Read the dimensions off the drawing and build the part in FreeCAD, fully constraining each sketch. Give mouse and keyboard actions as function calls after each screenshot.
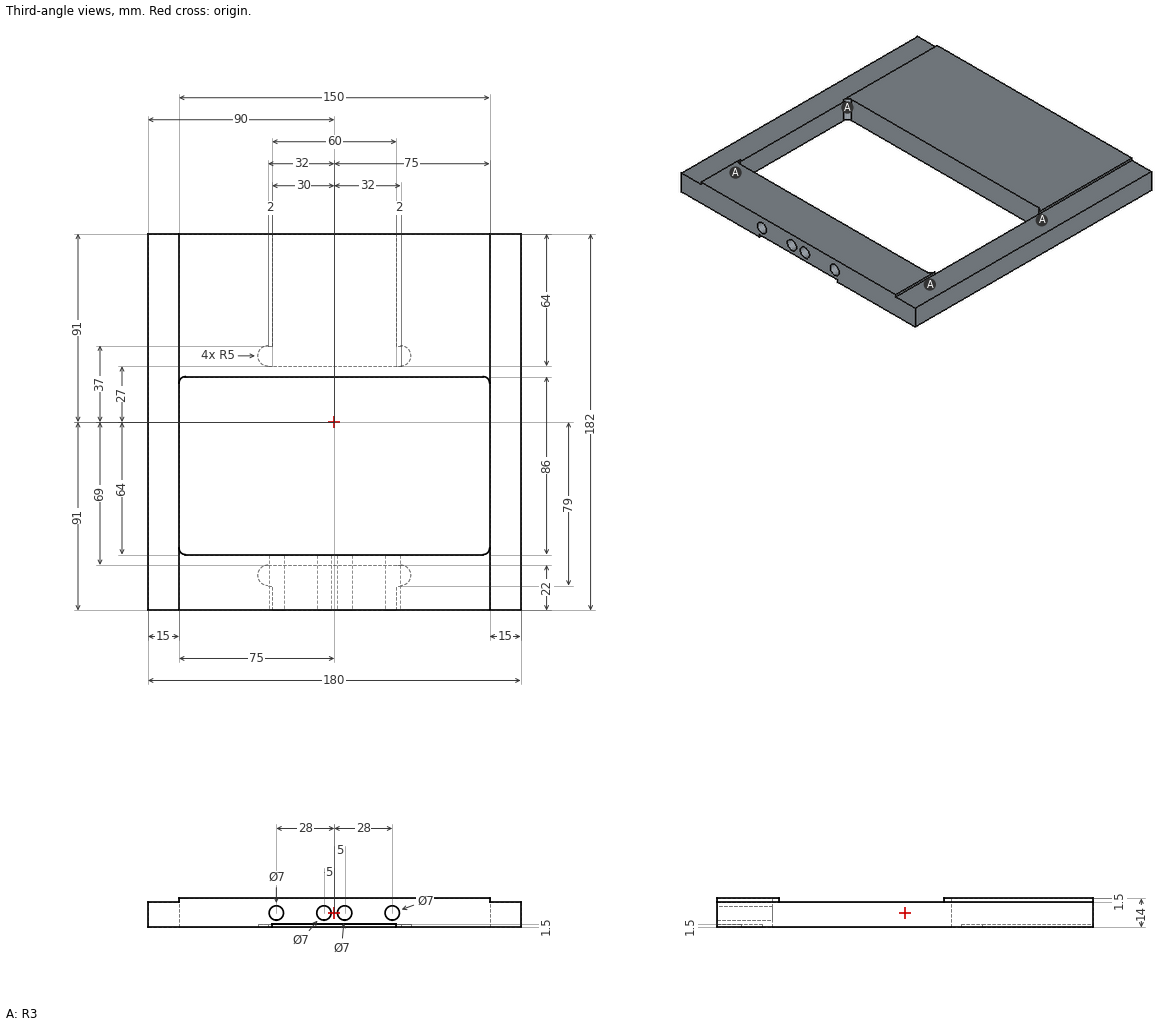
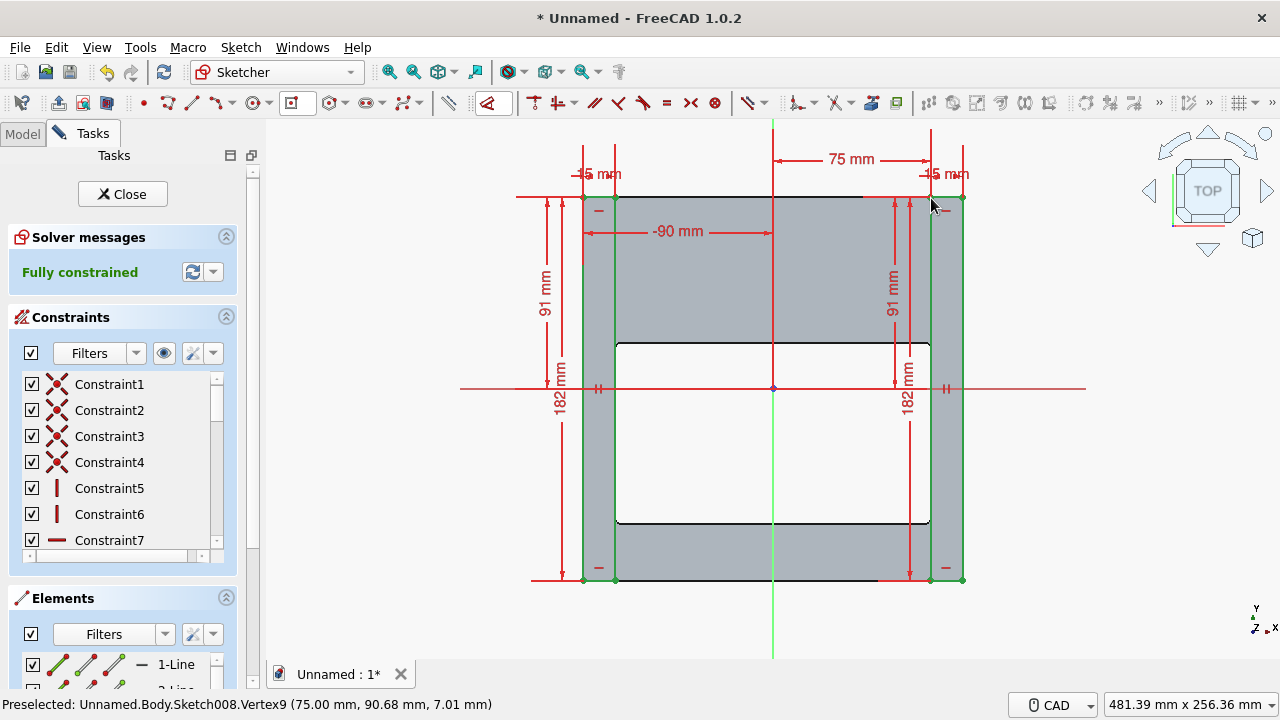
click(123, 194)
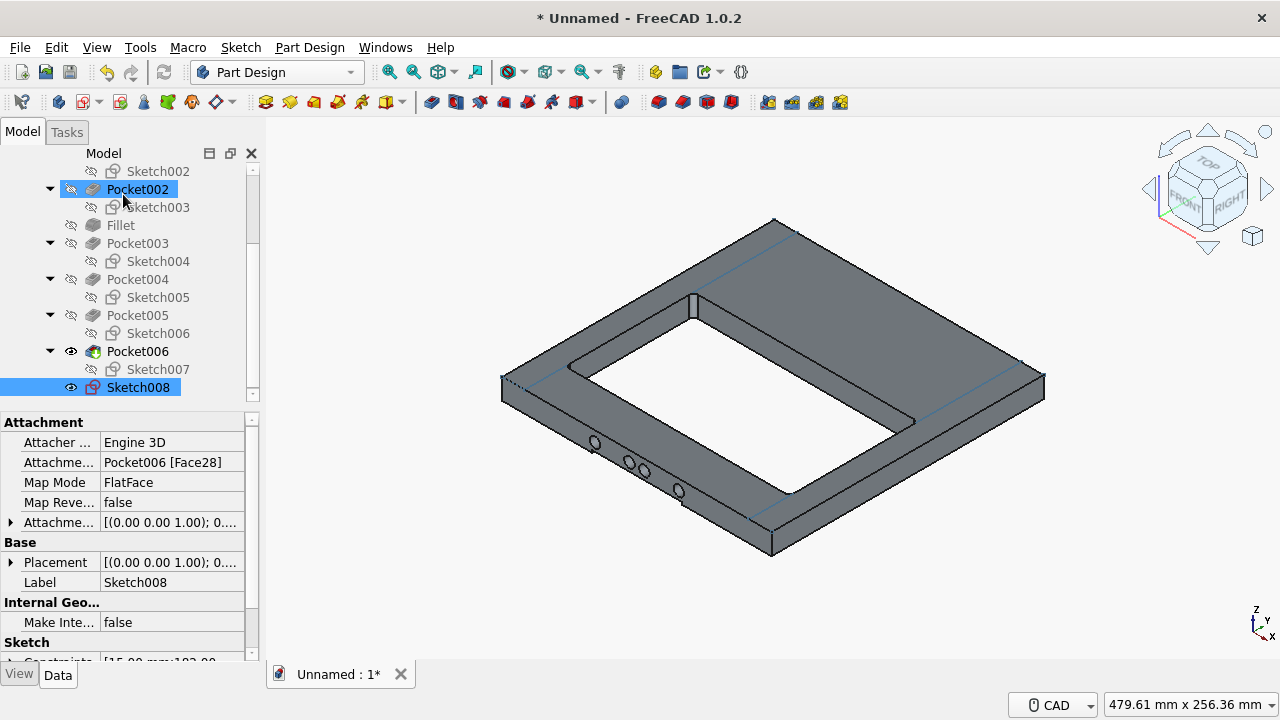
click(432, 102)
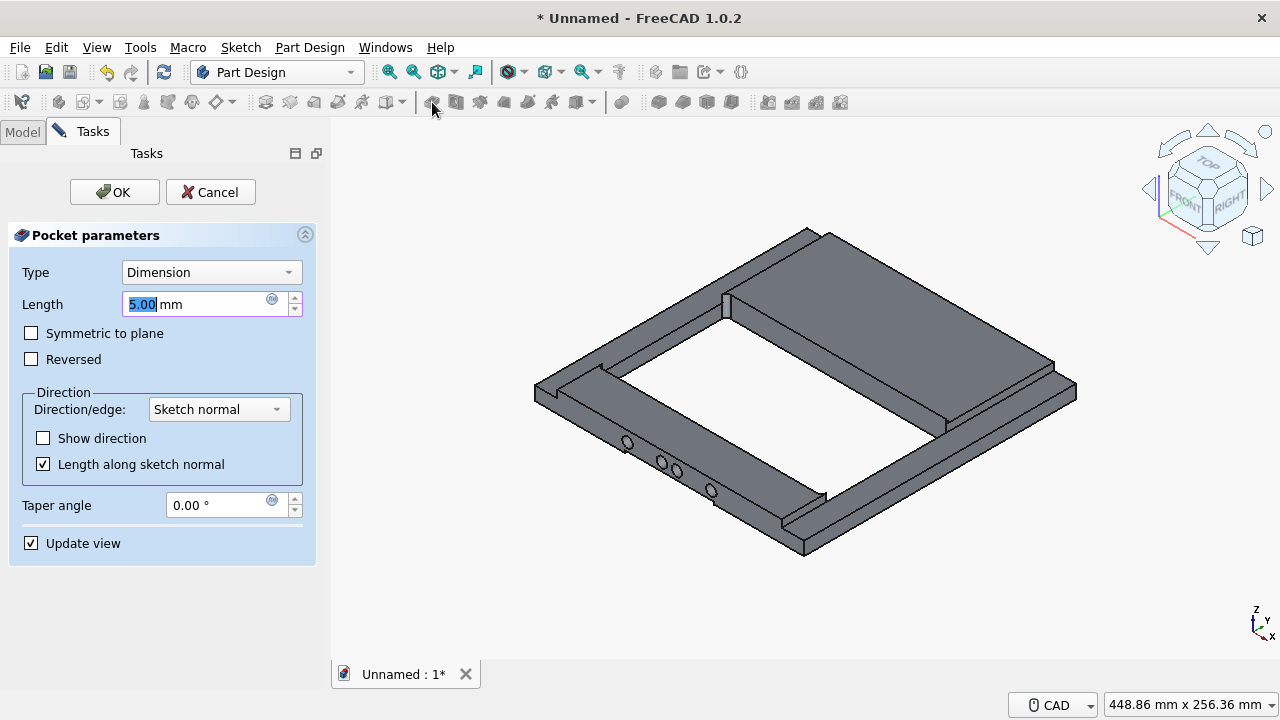
text(1.5)
key(Tab)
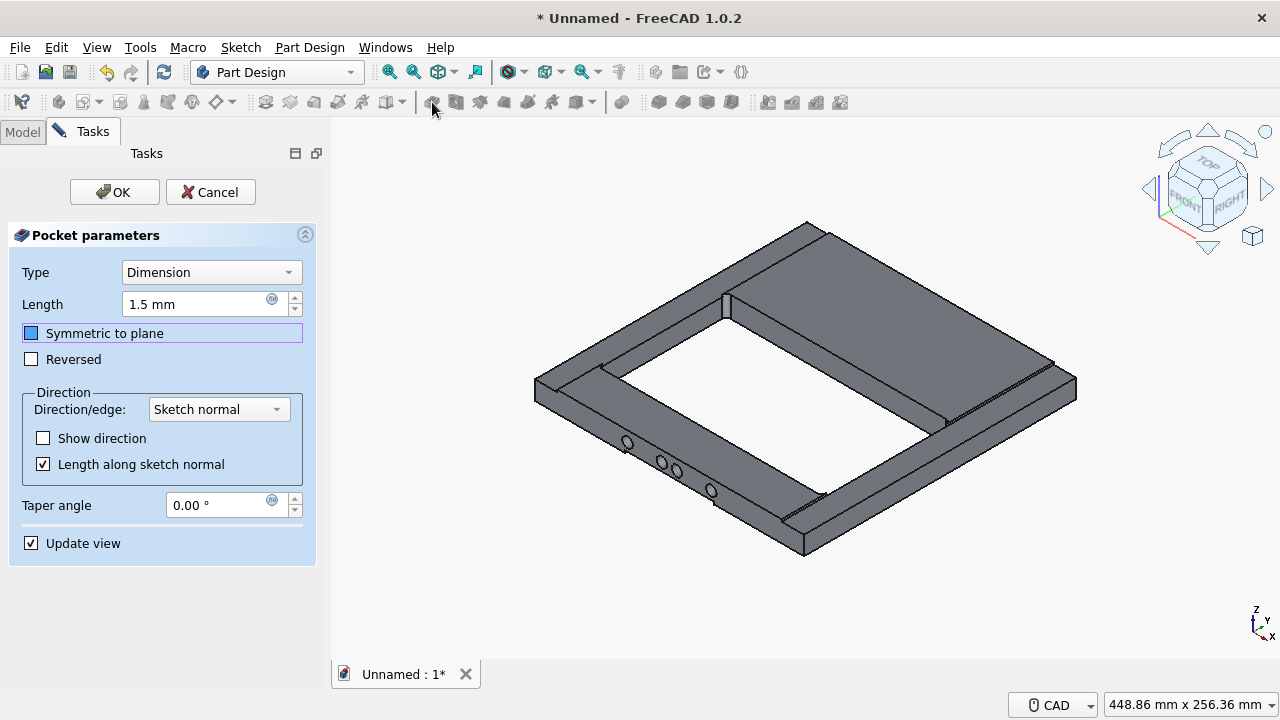
click(115, 192)